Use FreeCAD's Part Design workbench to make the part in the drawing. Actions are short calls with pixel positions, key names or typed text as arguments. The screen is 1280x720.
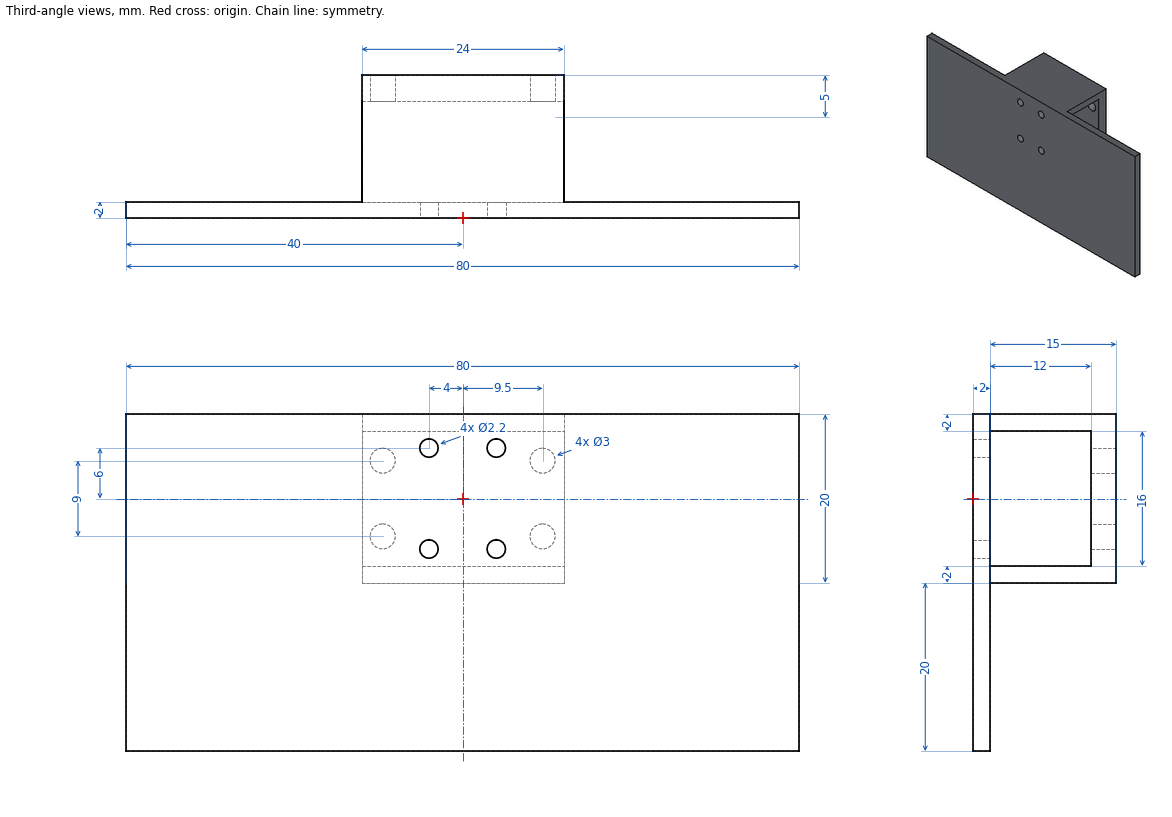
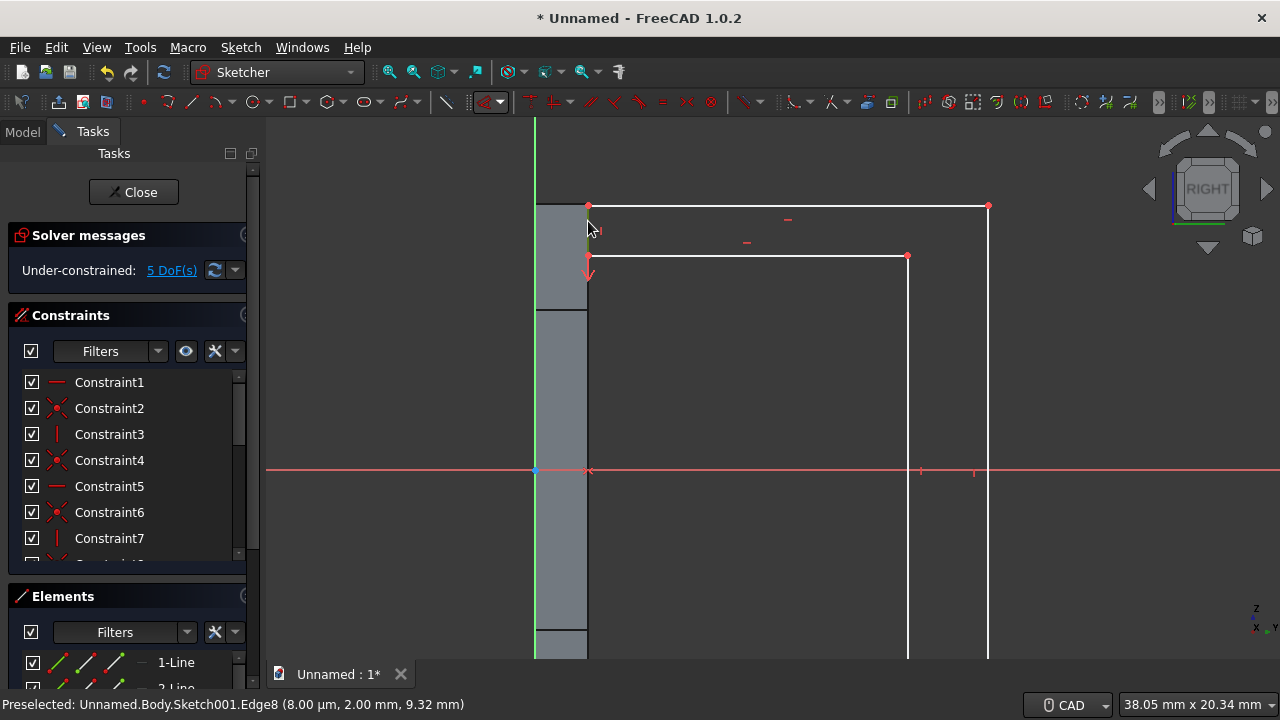
click(502, 102)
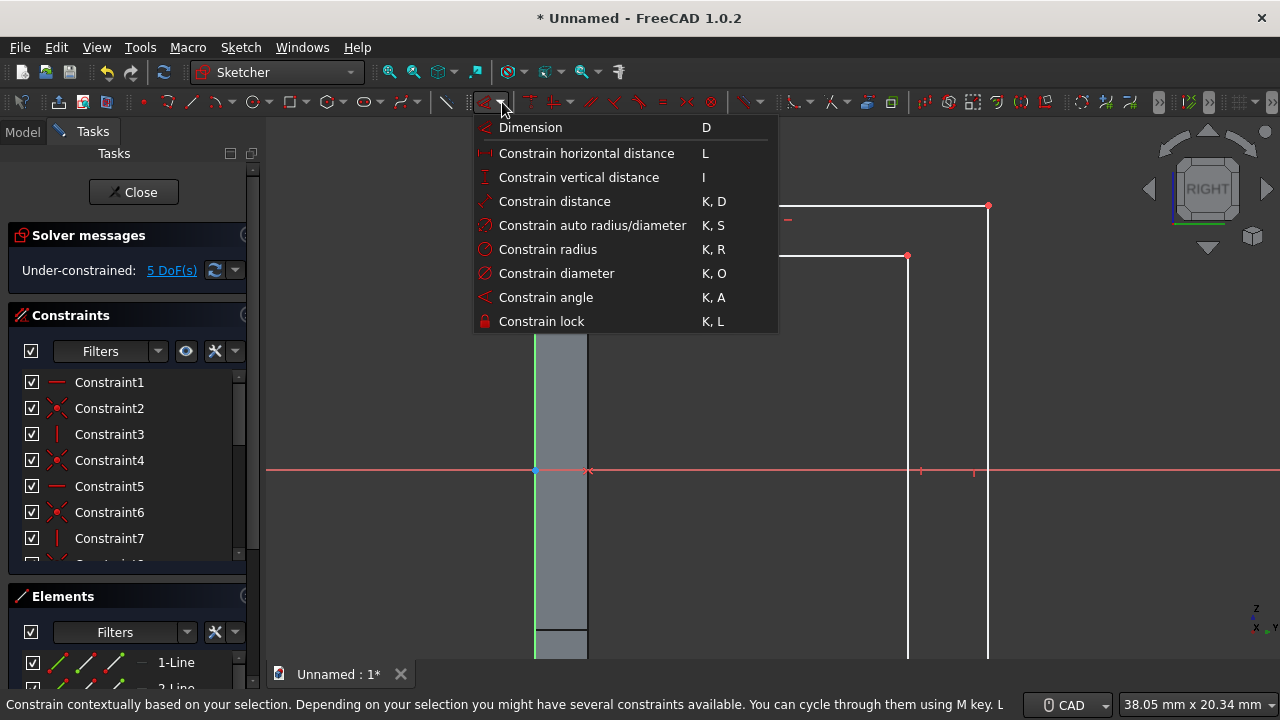
click(626, 177)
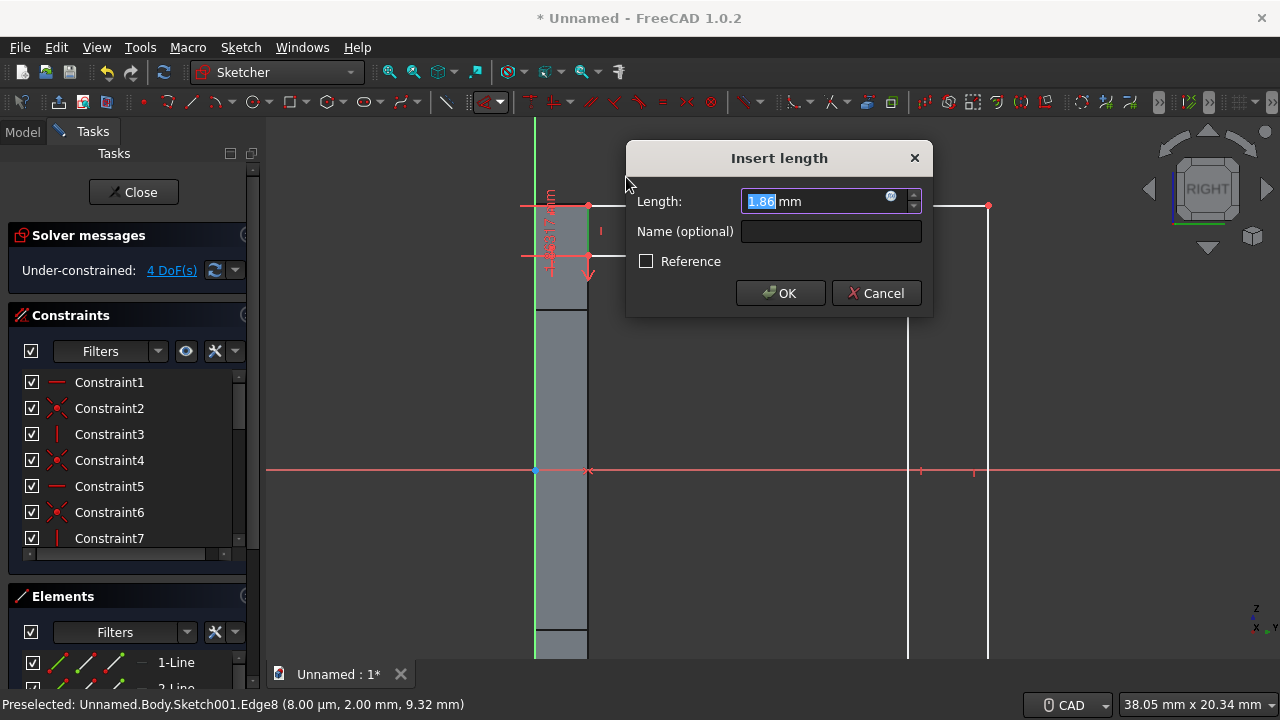
text(2)
key(Return)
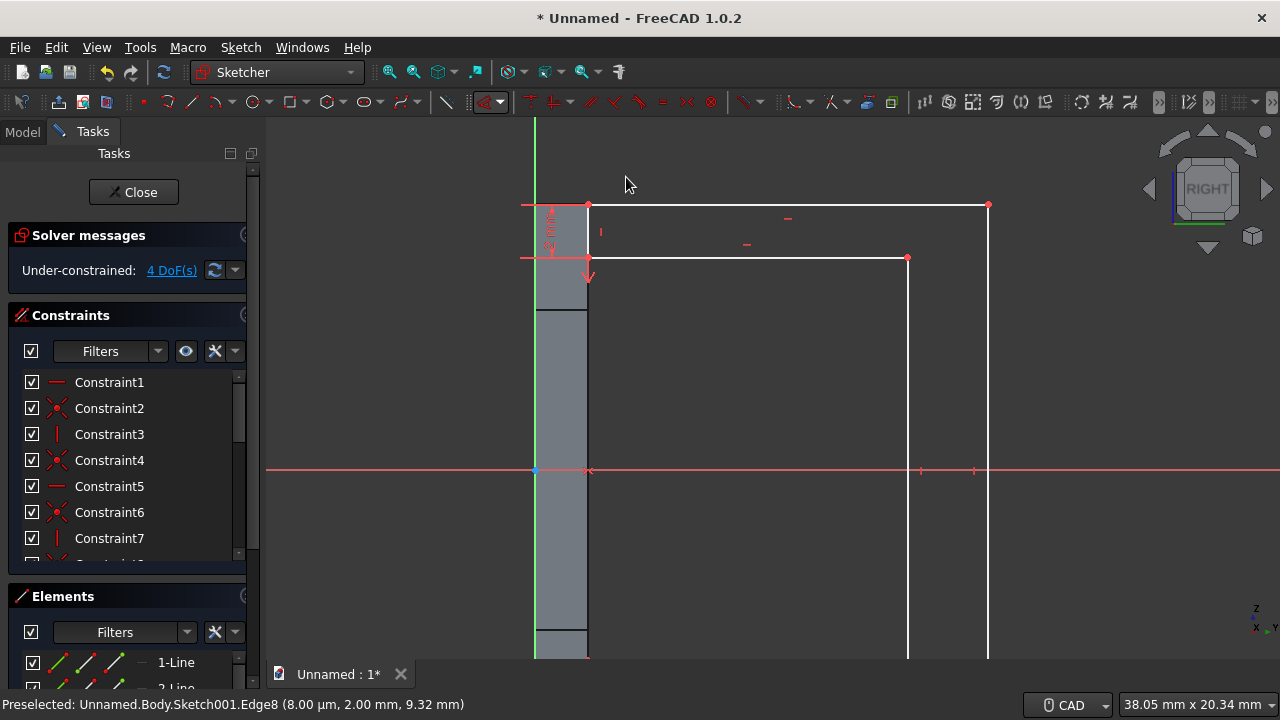
click(684, 258)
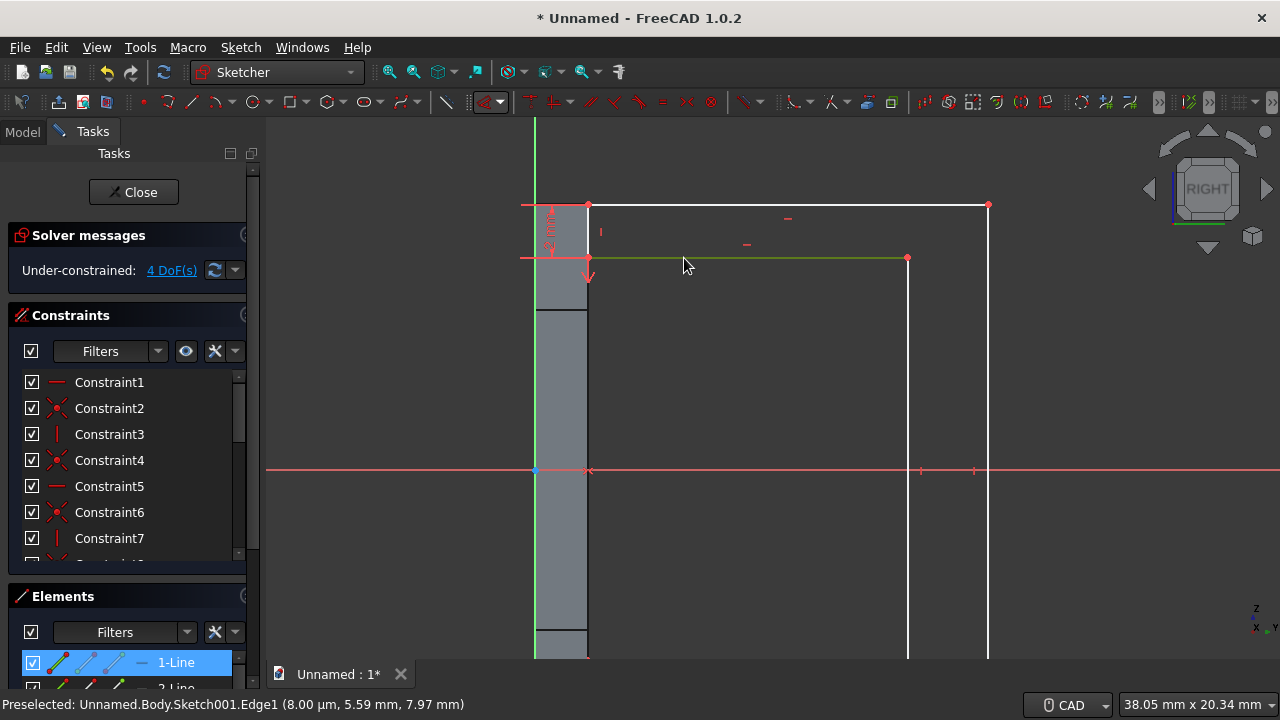
key(l)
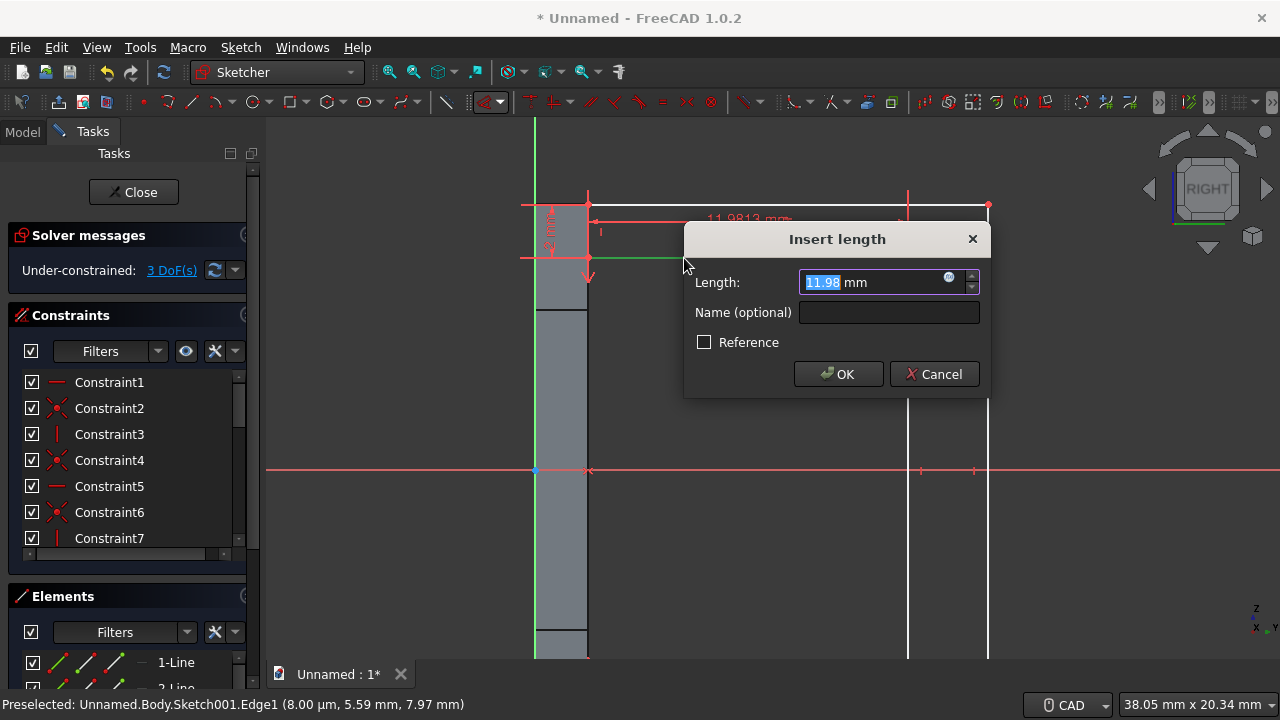
text(12)
key(Return)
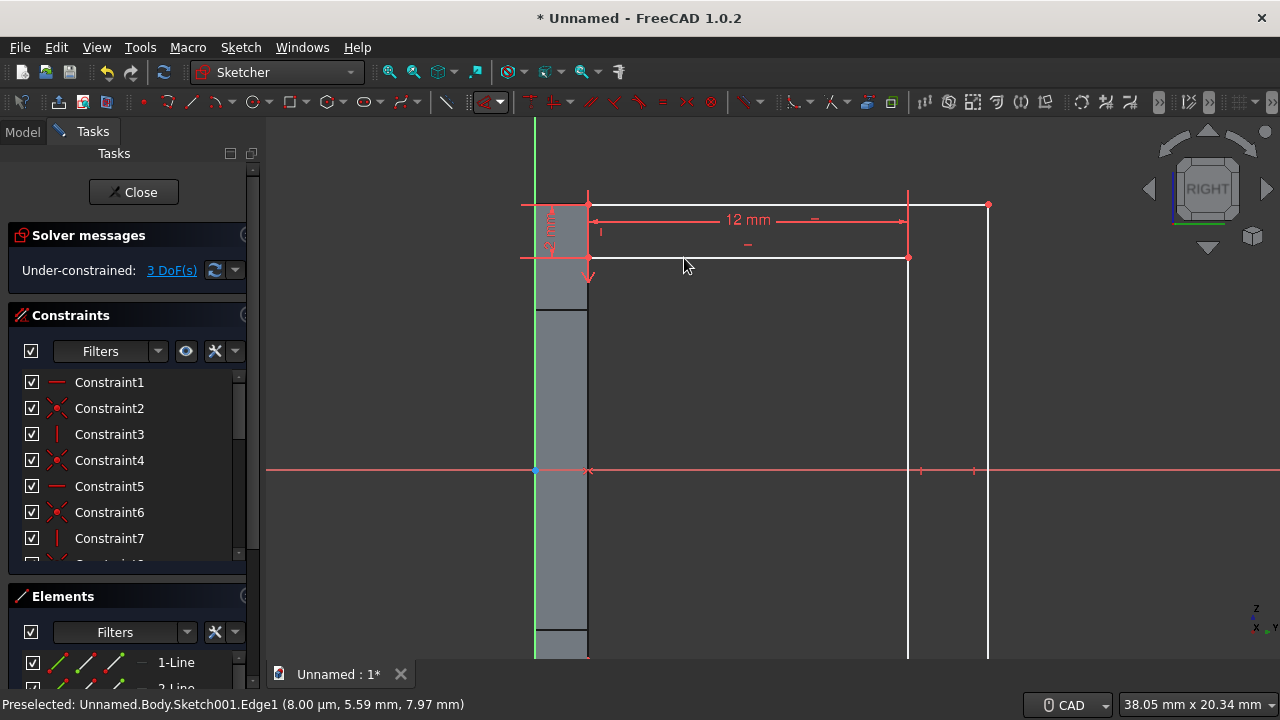
click(908, 385)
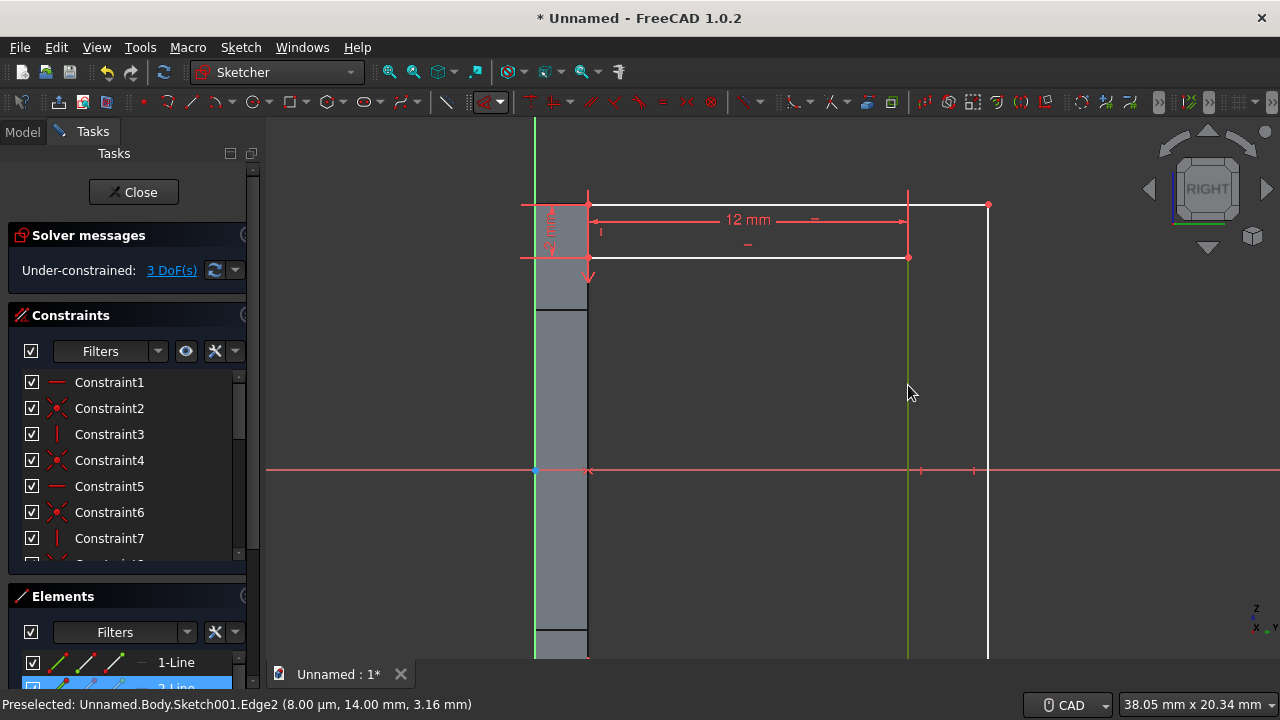
key(i)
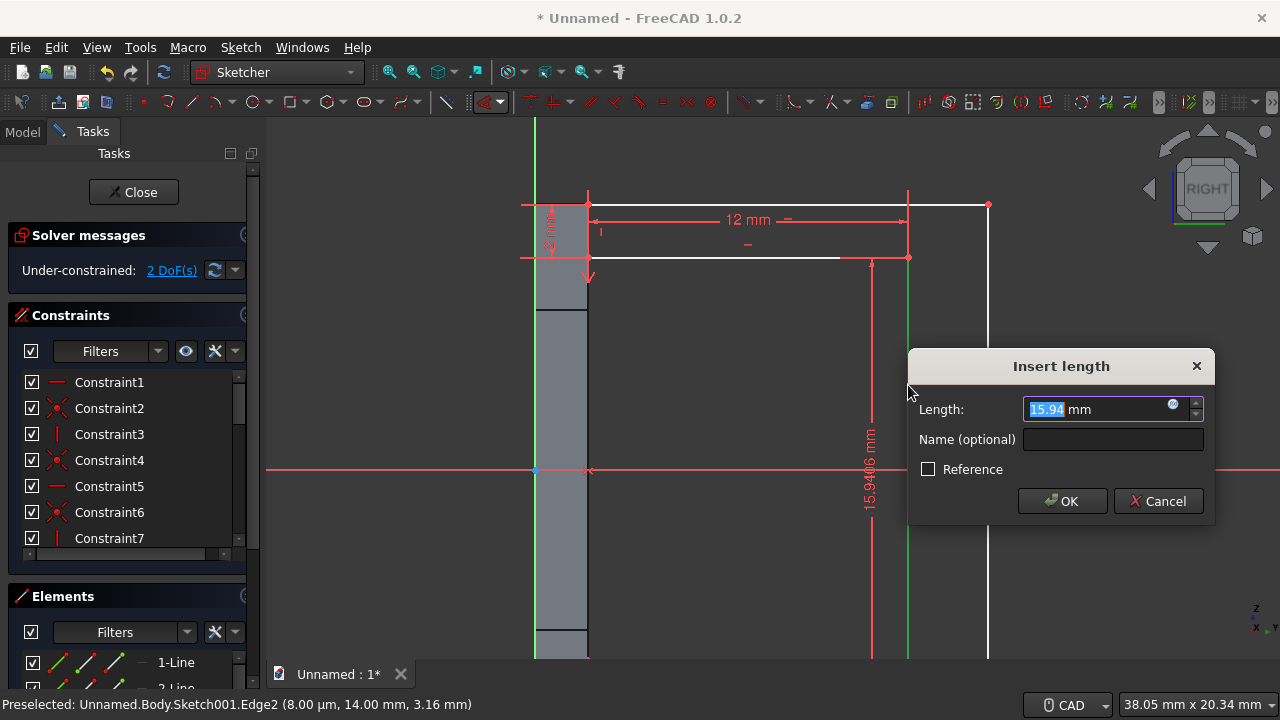
text(16)
key(Return)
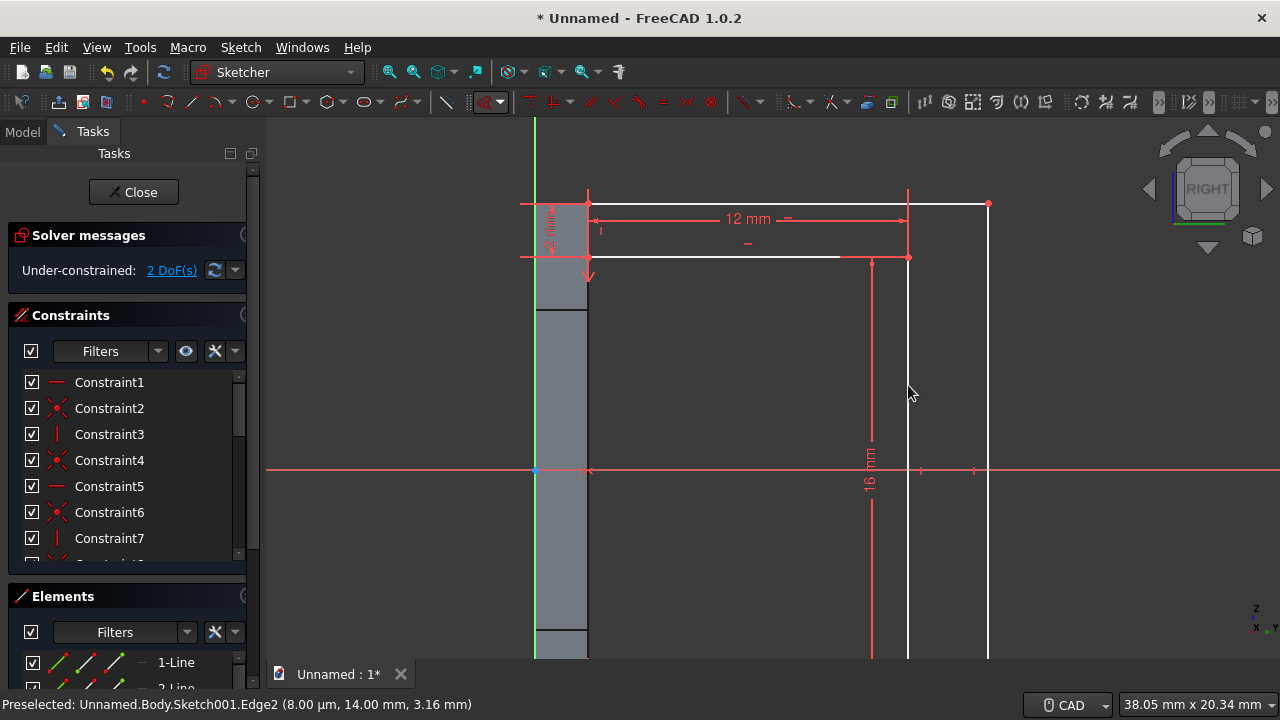
scroll(588, 221, down, 2)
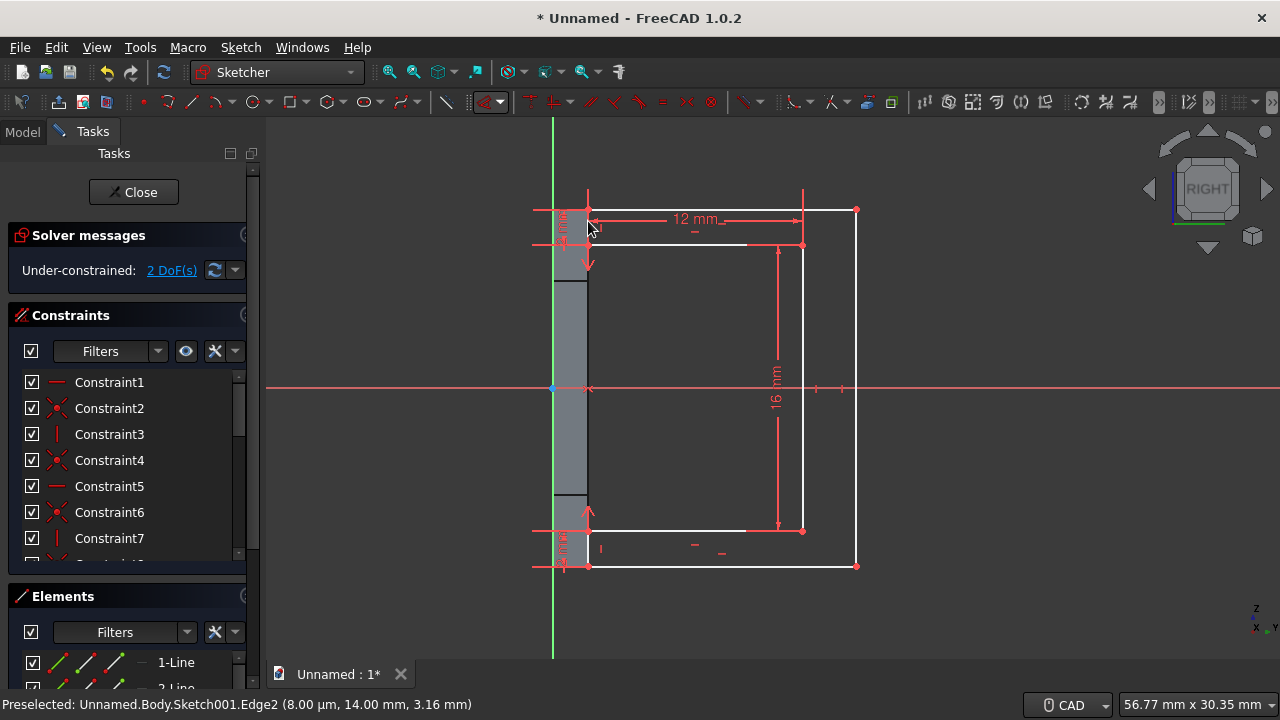
click(669, 567)